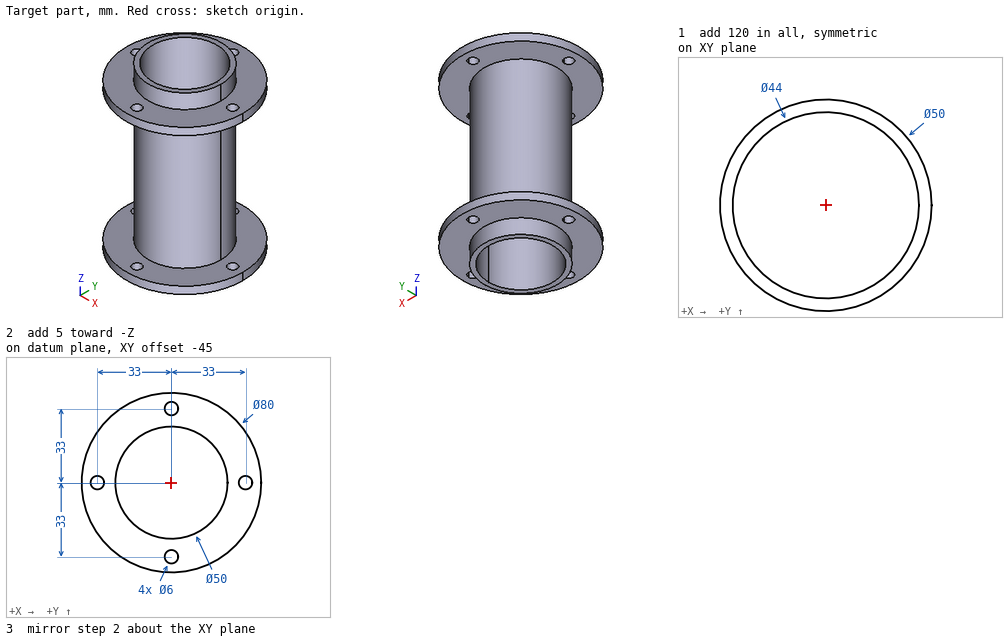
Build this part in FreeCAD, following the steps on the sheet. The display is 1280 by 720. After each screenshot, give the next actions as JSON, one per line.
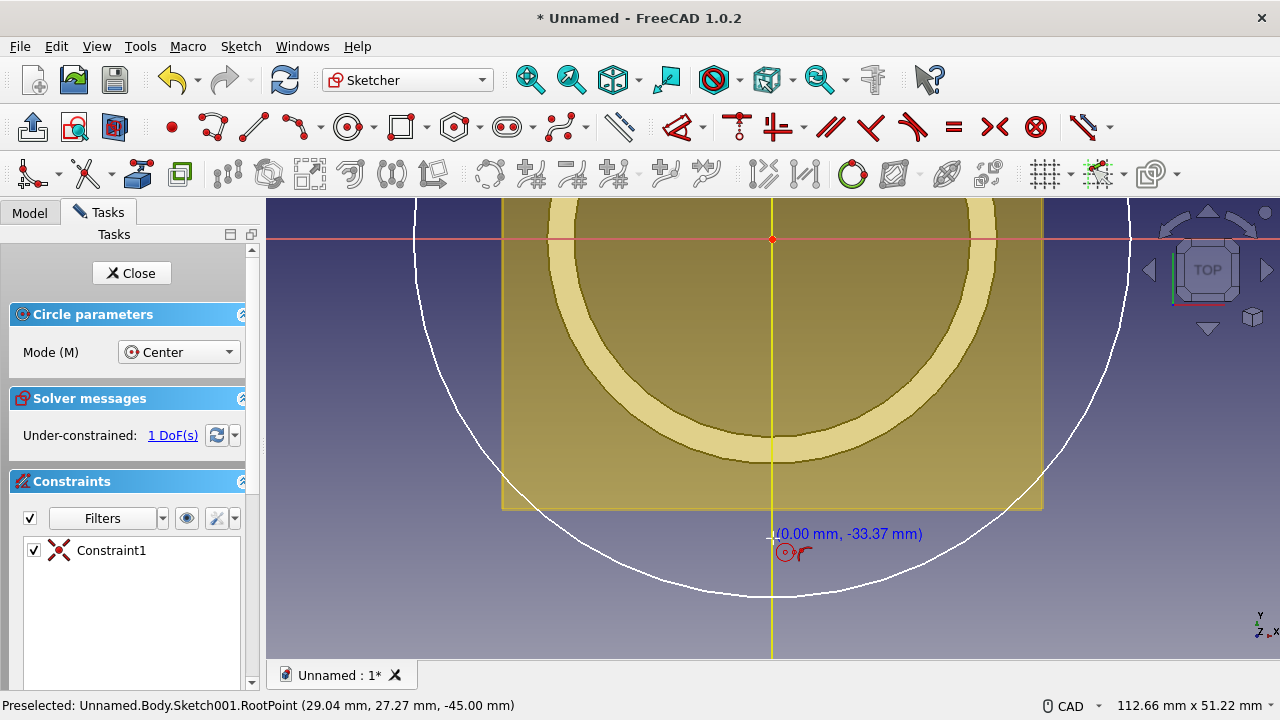
{"action": "left_click", "coordinate": [772, 536]}
{"action": "left_click", "coordinate": [791, 517]}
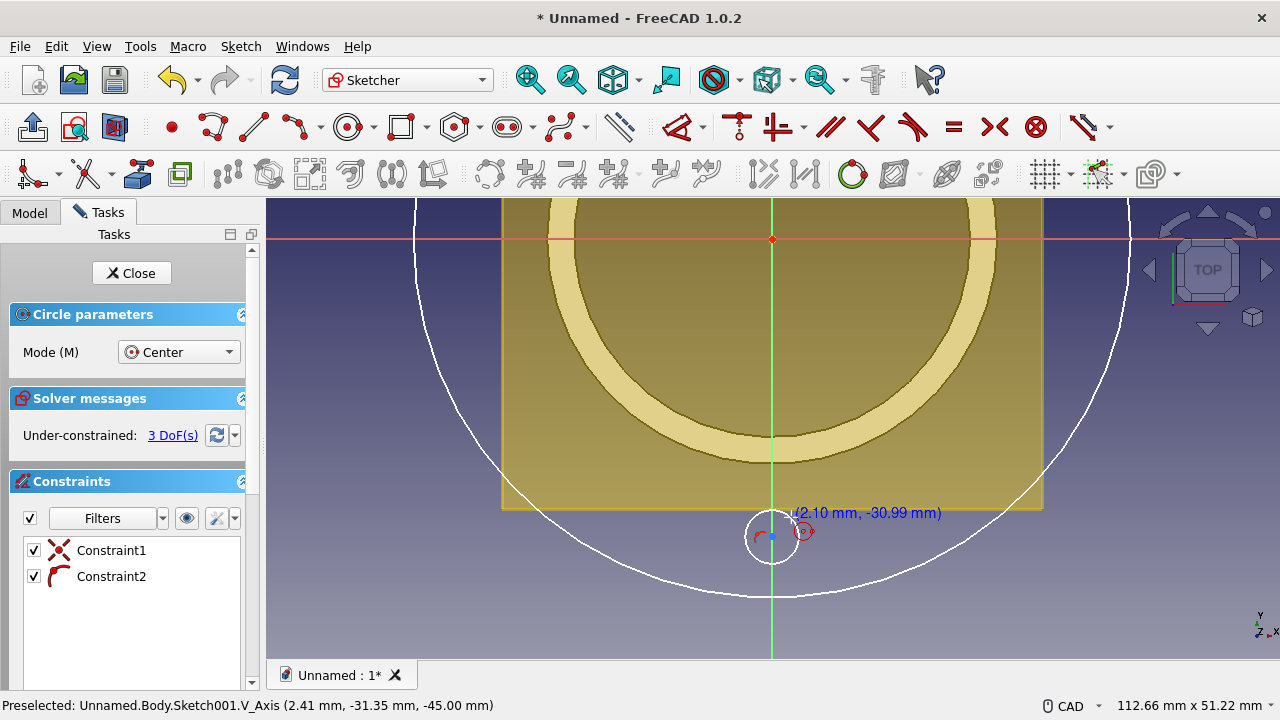
{"action": "left_click", "coordinate": [1069, 239]}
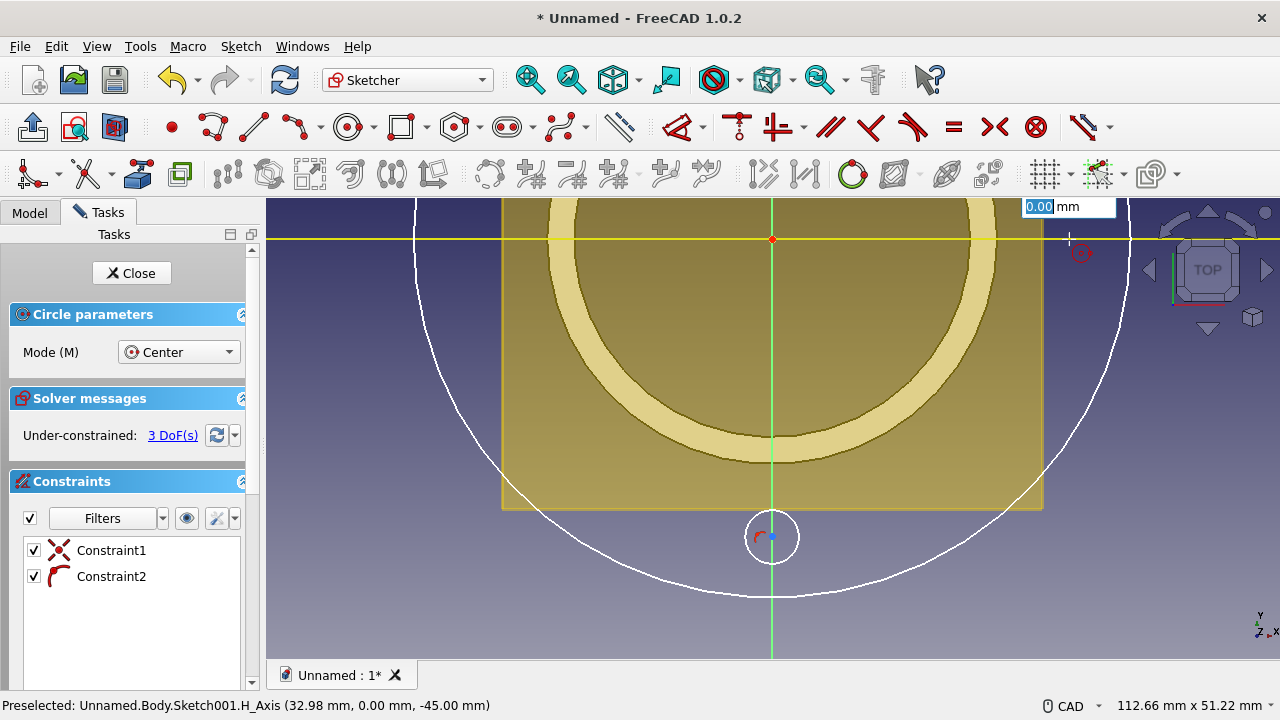
{"action": "scroll", "coordinate": [665, 539], "scroll_direction": "down", "scroll_amount": 5}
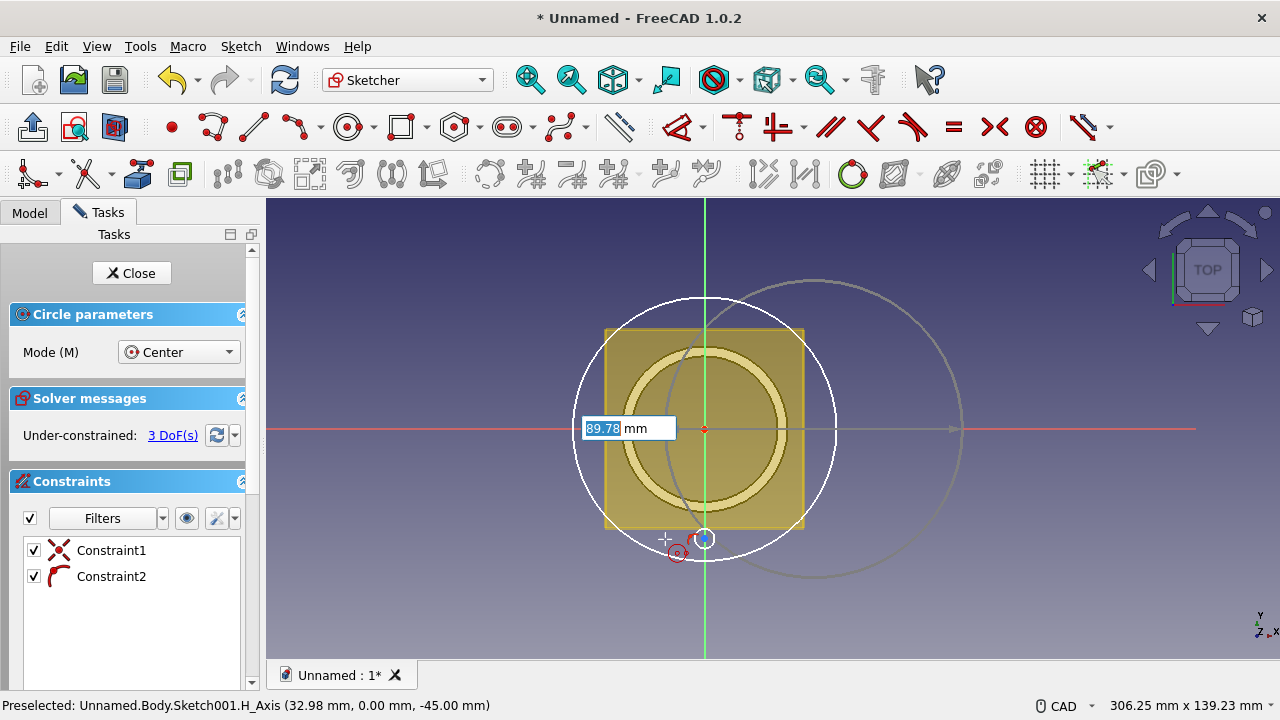
{"action": "scroll", "coordinate": [821, 422], "scroll_direction": "up", "scroll_amount": 5}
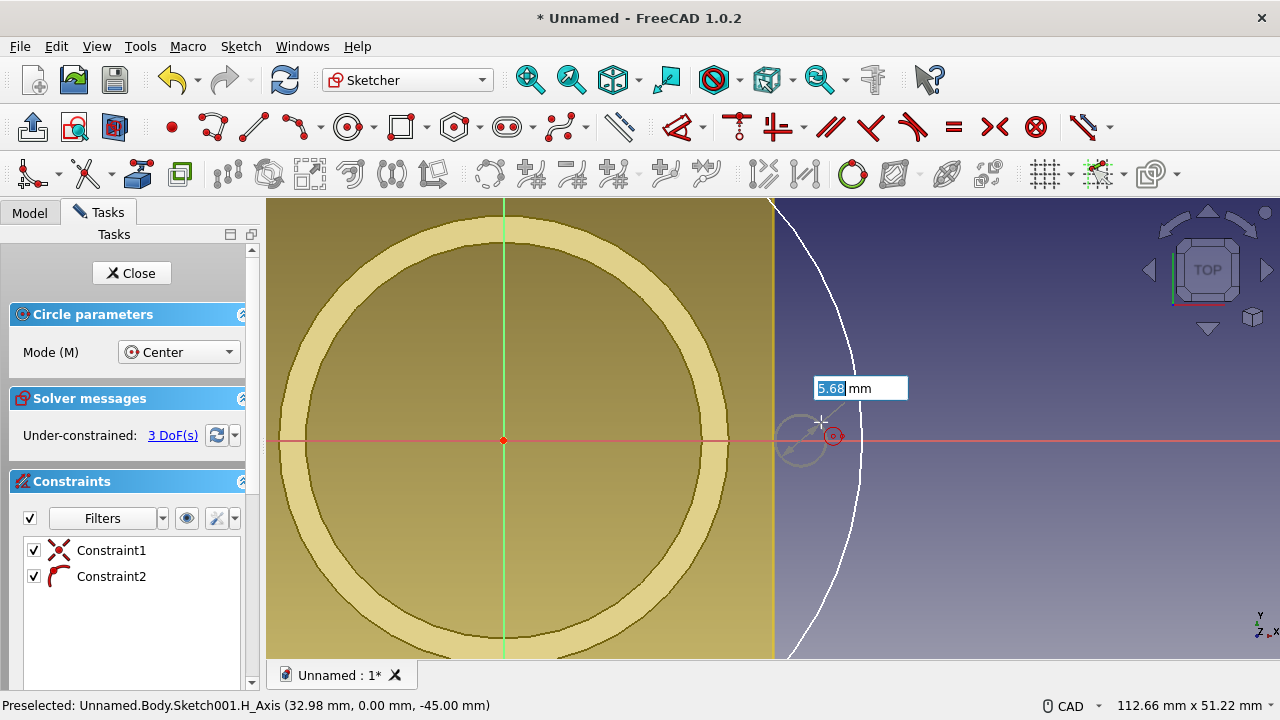
{"action": "left_click", "coordinate": [820, 421]}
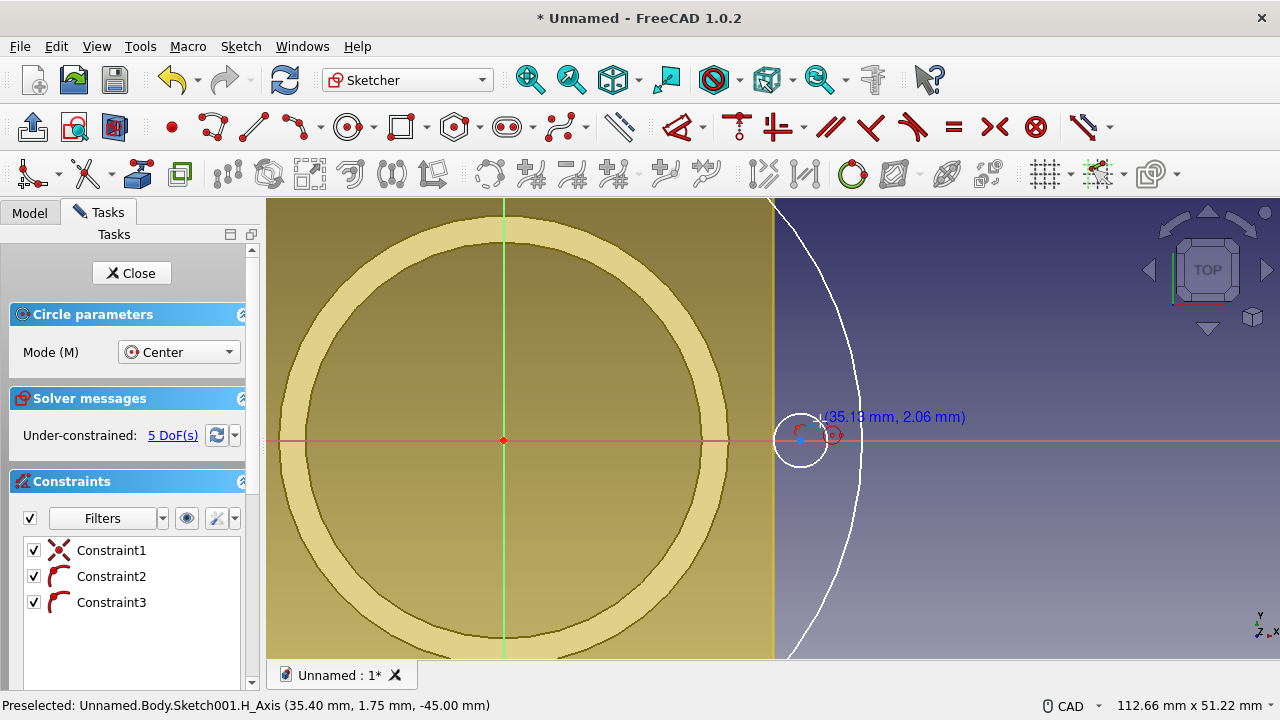
{"action": "left_click", "coordinate": [504, 441]}
{"action": "left_click", "coordinate": [663, 281]}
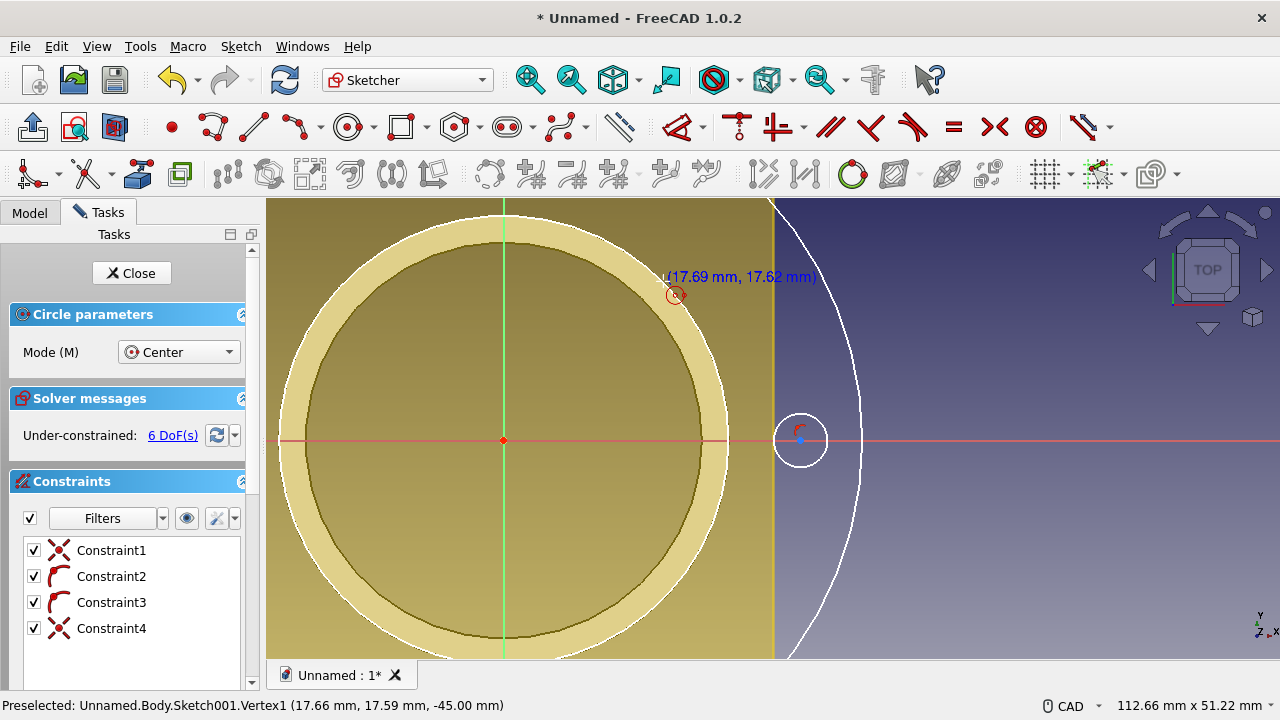
{"action": "scroll", "coordinate": [821, 421], "scroll_direction": "down", "scroll_amount": 5}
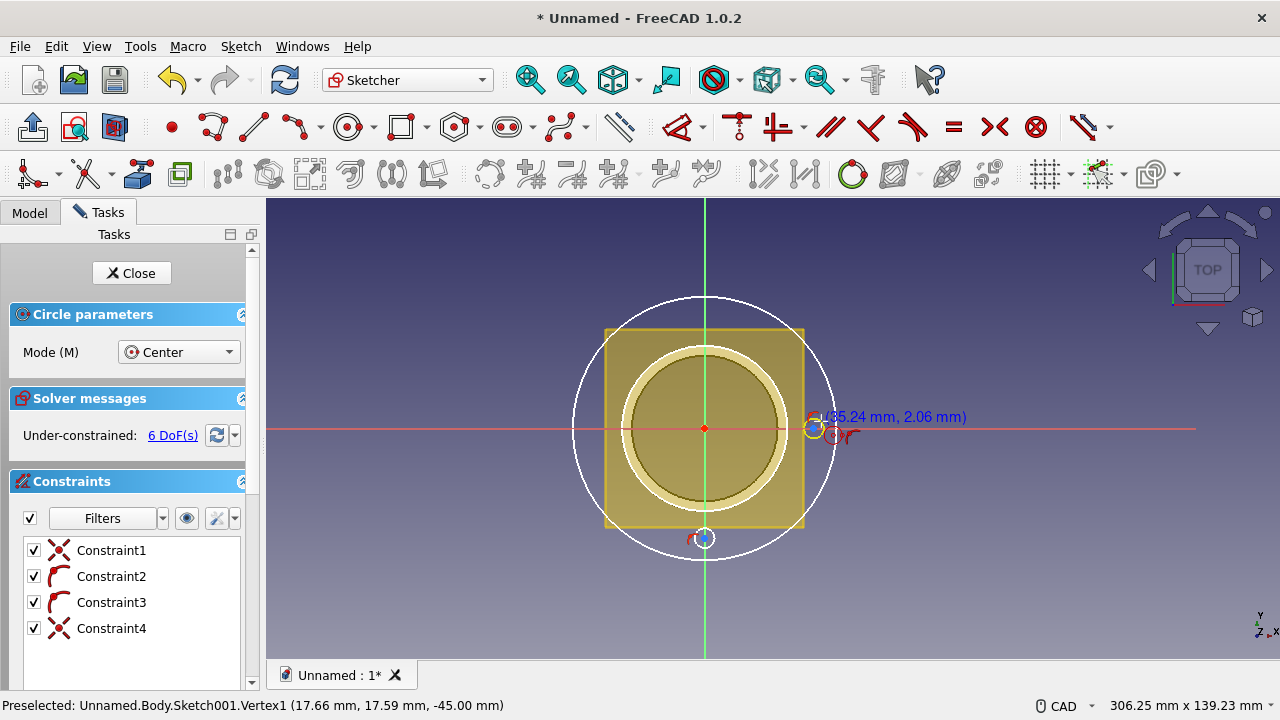
{"action": "scroll", "coordinate": [595, 428], "scroll_direction": "up", "scroll_amount": 5}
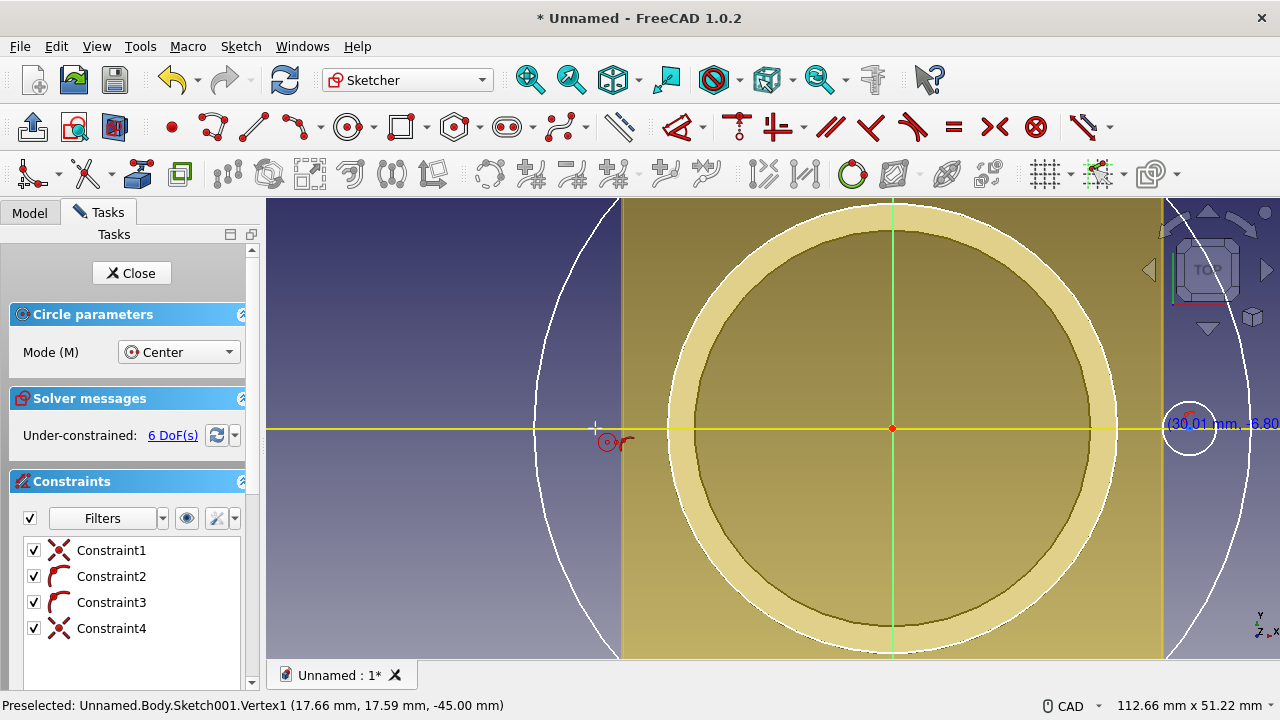
{"action": "left_click", "coordinate": [596, 428]}
{"action": "left_click", "coordinate": [615, 409]}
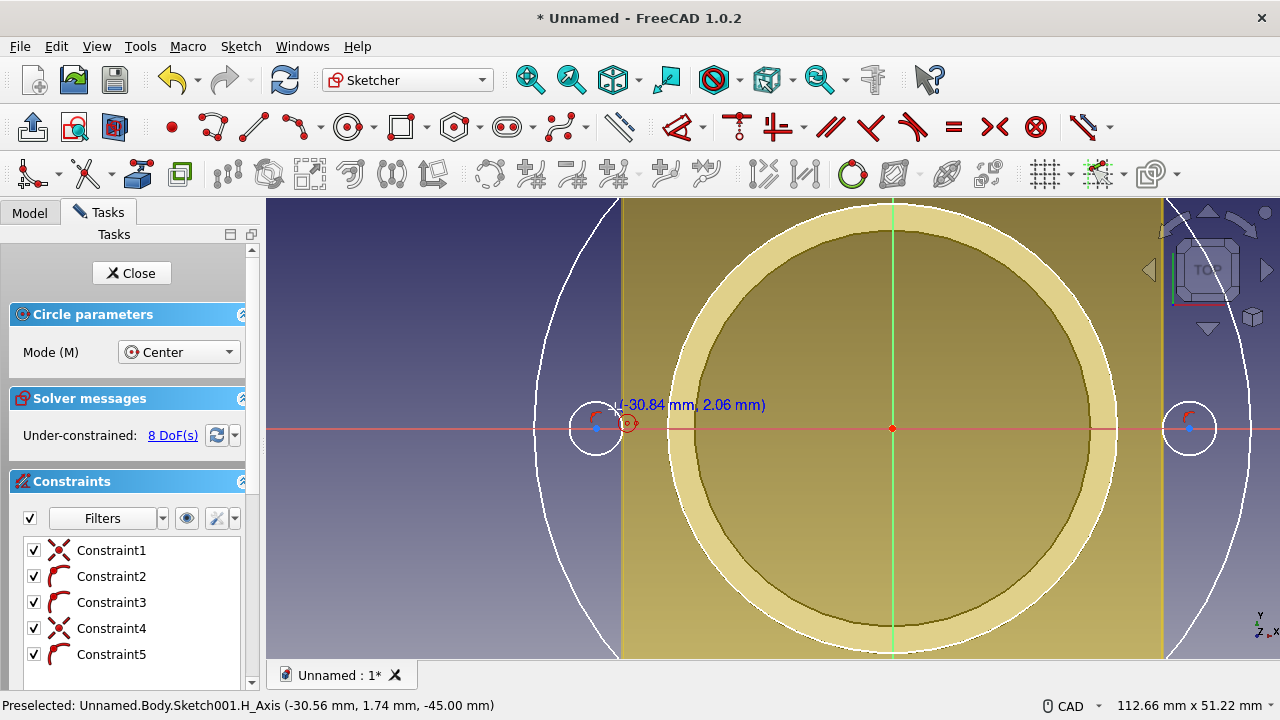
{"action": "scroll", "coordinate": [595, 429], "scroll_direction": "down", "scroll_amount": 5}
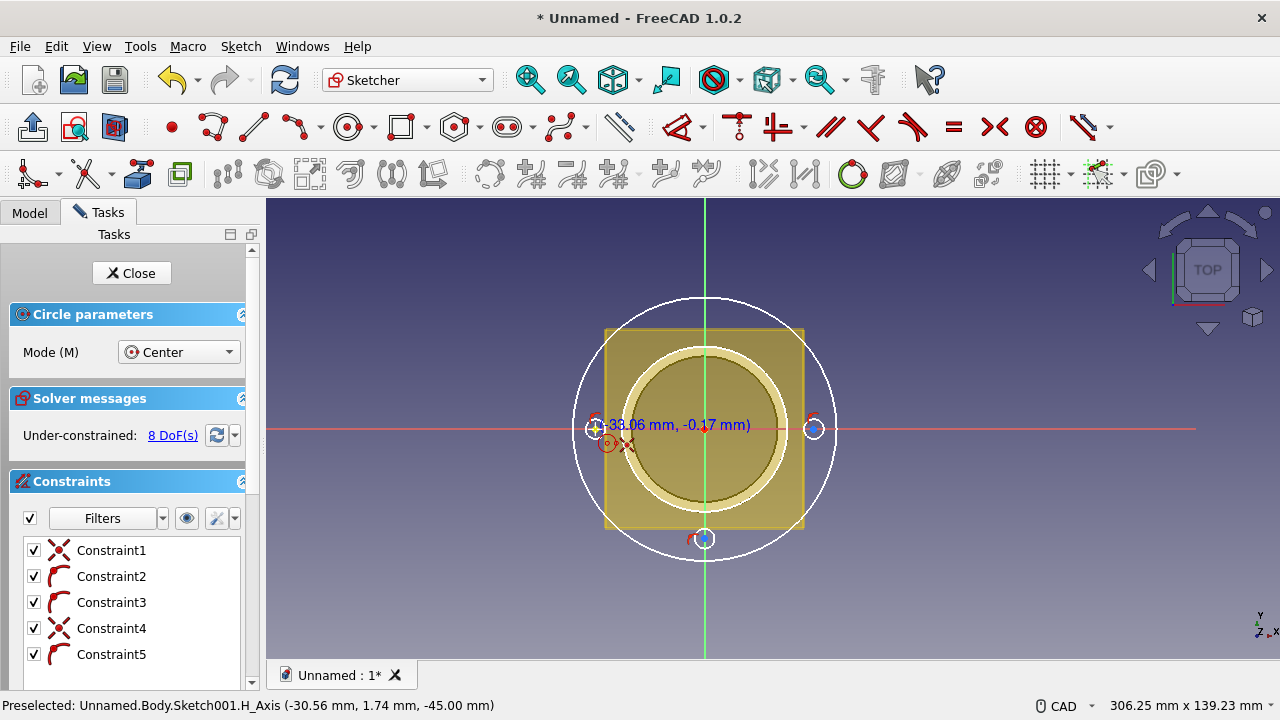
{"action": "scroll", "coordinate": [705, 320], "scroll_direction": "up", "scroll_amount": 5}